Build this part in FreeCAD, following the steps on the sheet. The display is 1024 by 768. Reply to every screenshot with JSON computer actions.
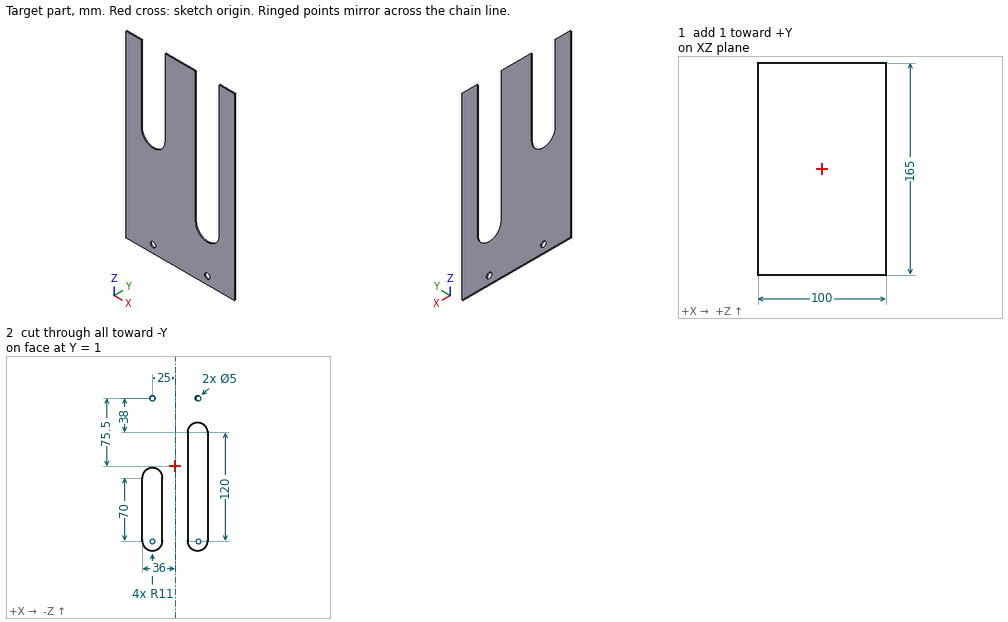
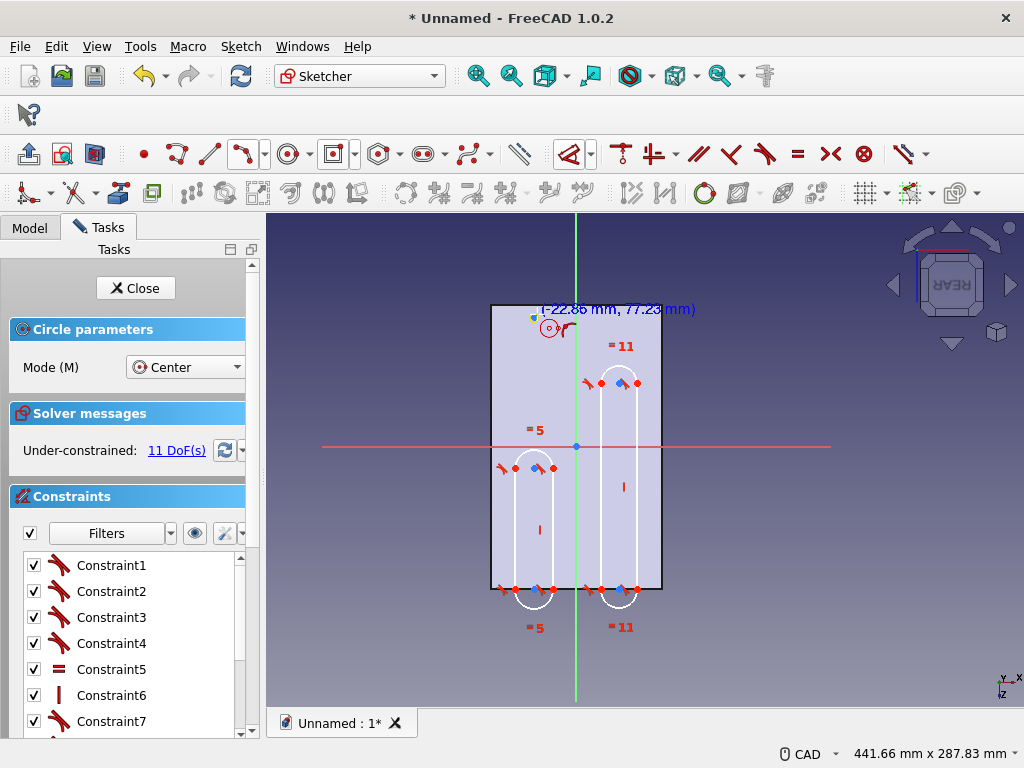
{"action": "scroll", "coordinate": [619, 317], "scroll_direction": "up", "scroll_amount": 9}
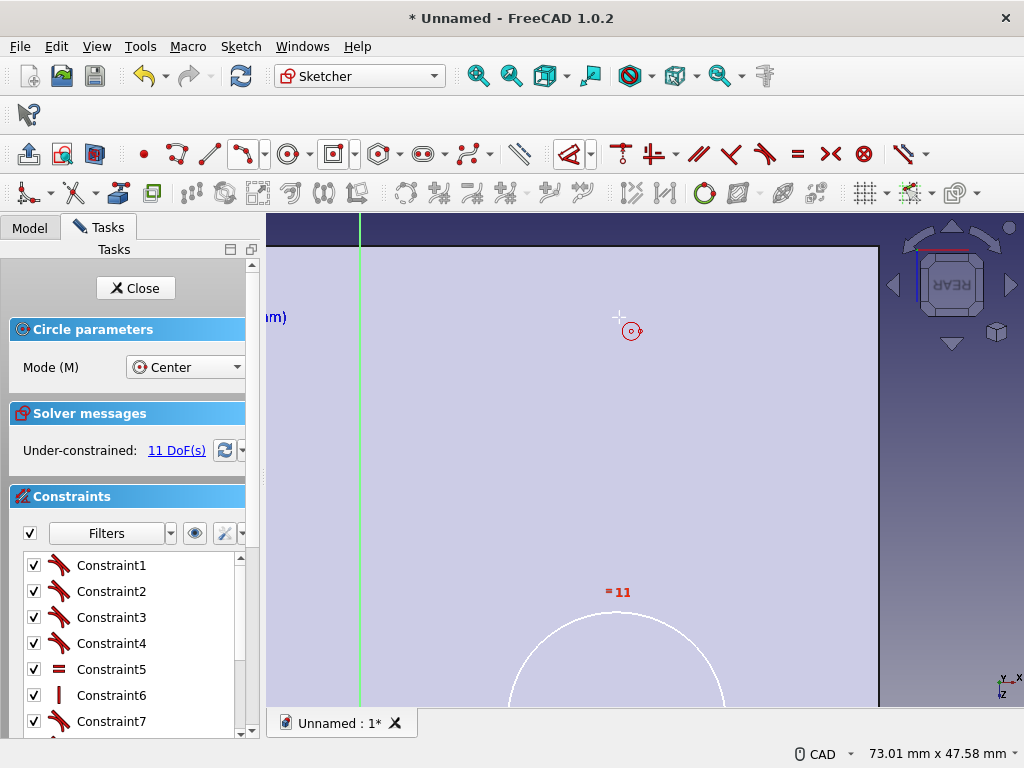
{"action": "scroll", "coordinate": [619, 317], "scroll_direction": "down", "scroll_amount": 9}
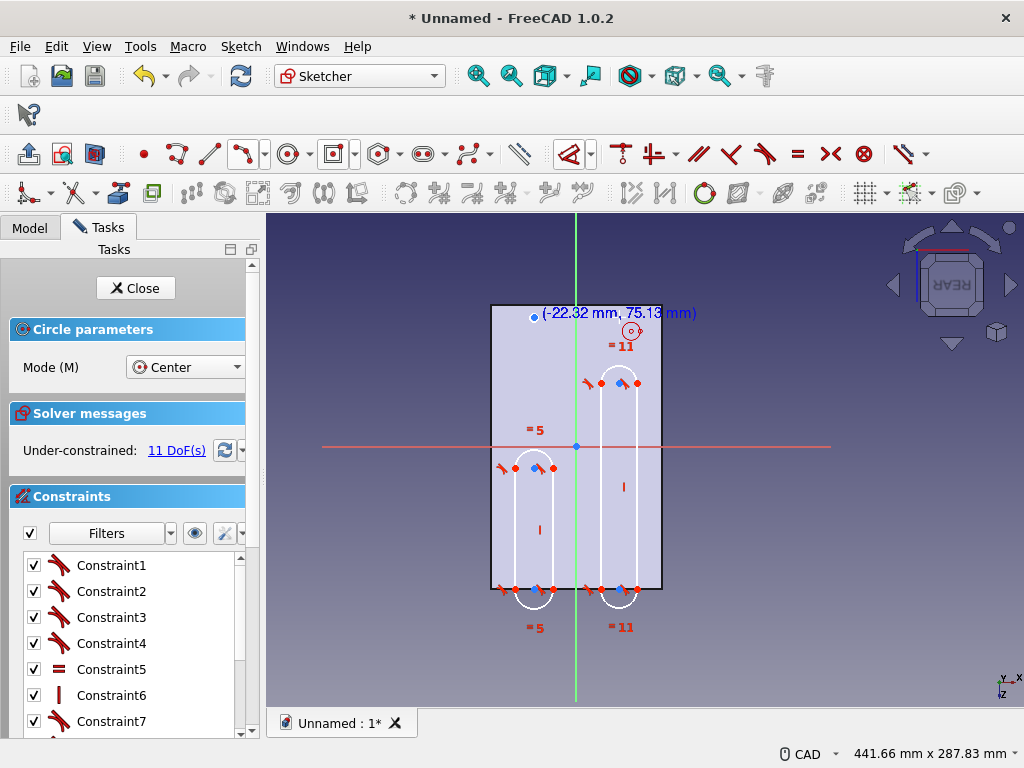
{"action": "left_click", "coordinate": [619, 317]}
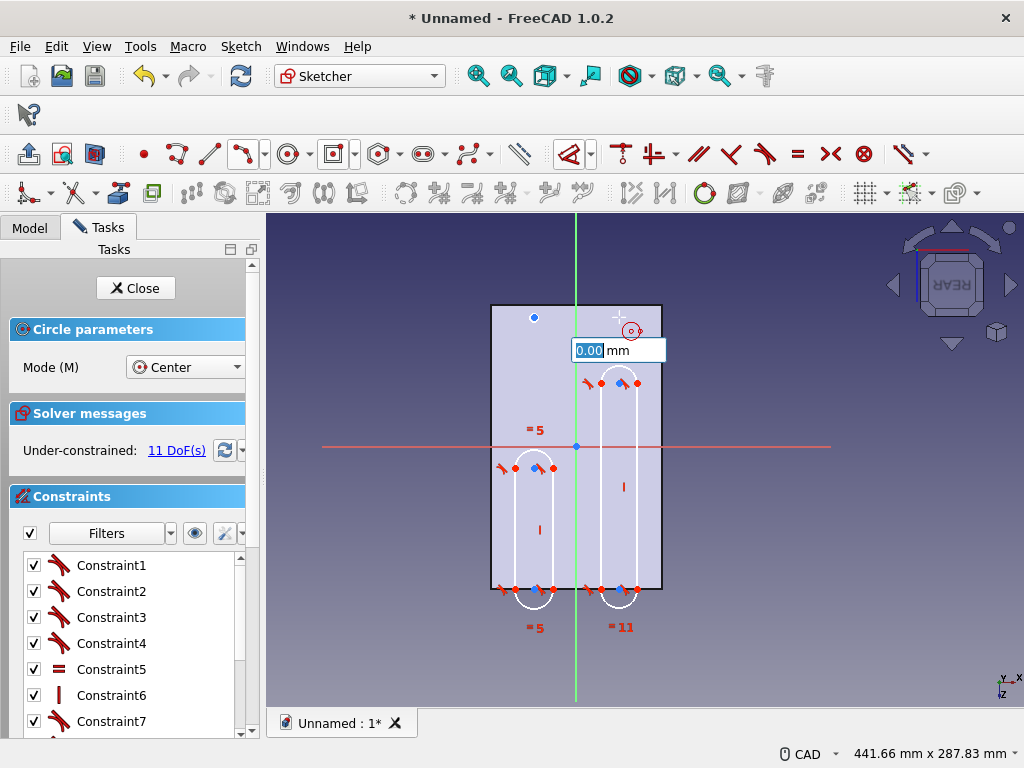
{"action": "scroll", "coordinate": [622, 314], "scroll_direction": "up", "scroll_amount": 7}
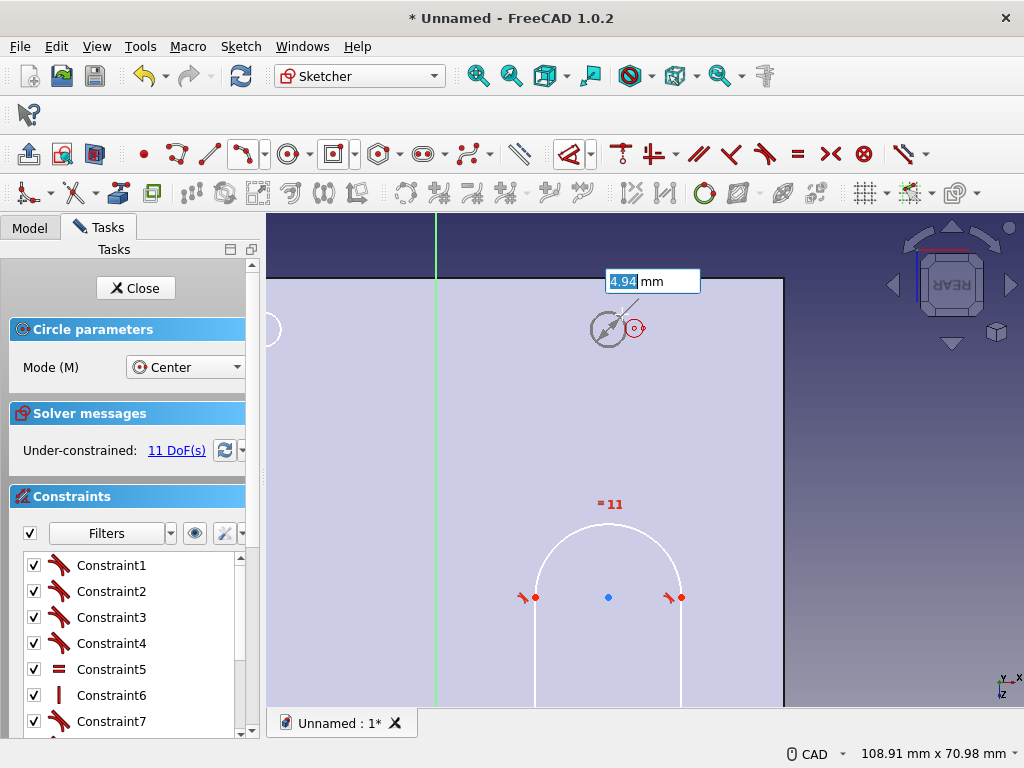
{"action": "left_click", "coordinate": [622, 315]}
{"action": "key", "text": "Escape"}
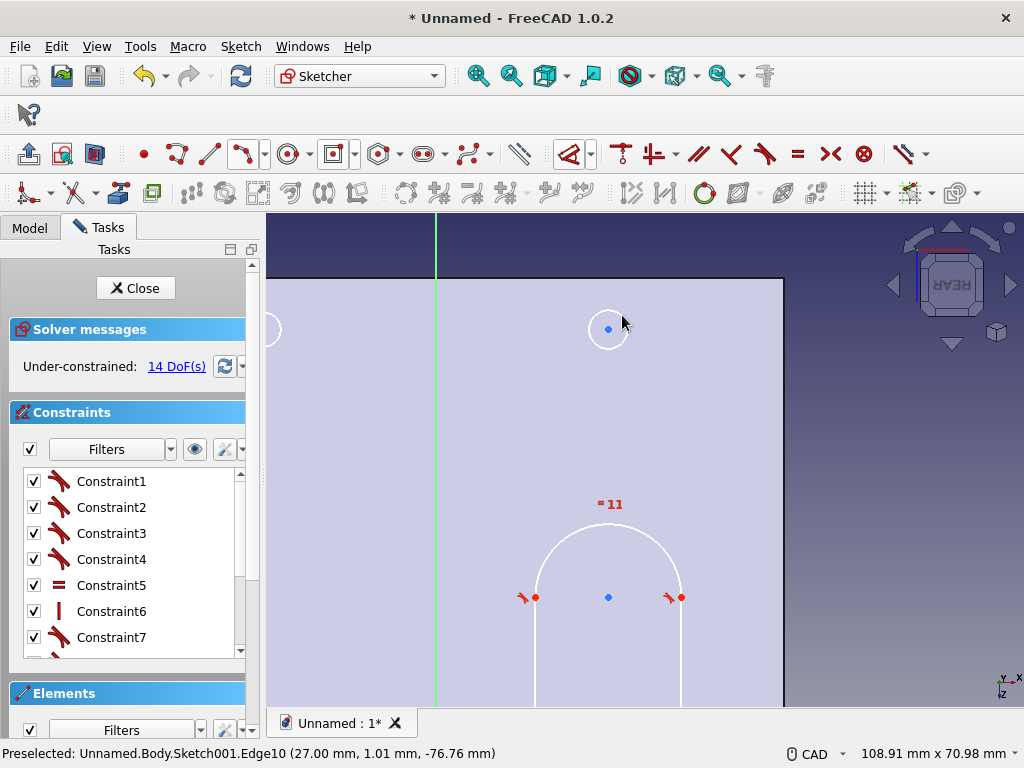
{"action": "scroll", "coordinate": [622, 314], "scroll_direction": "down", "scroll_amount": 7}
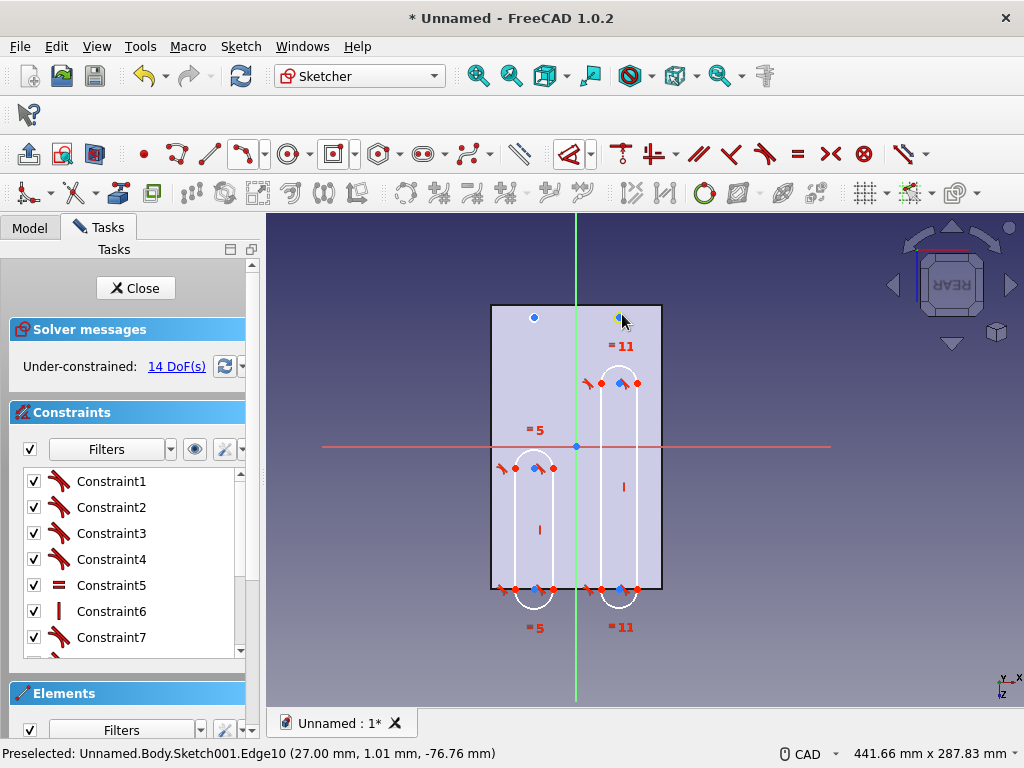
{"action": "left_click", "coordinate": [523, 605]}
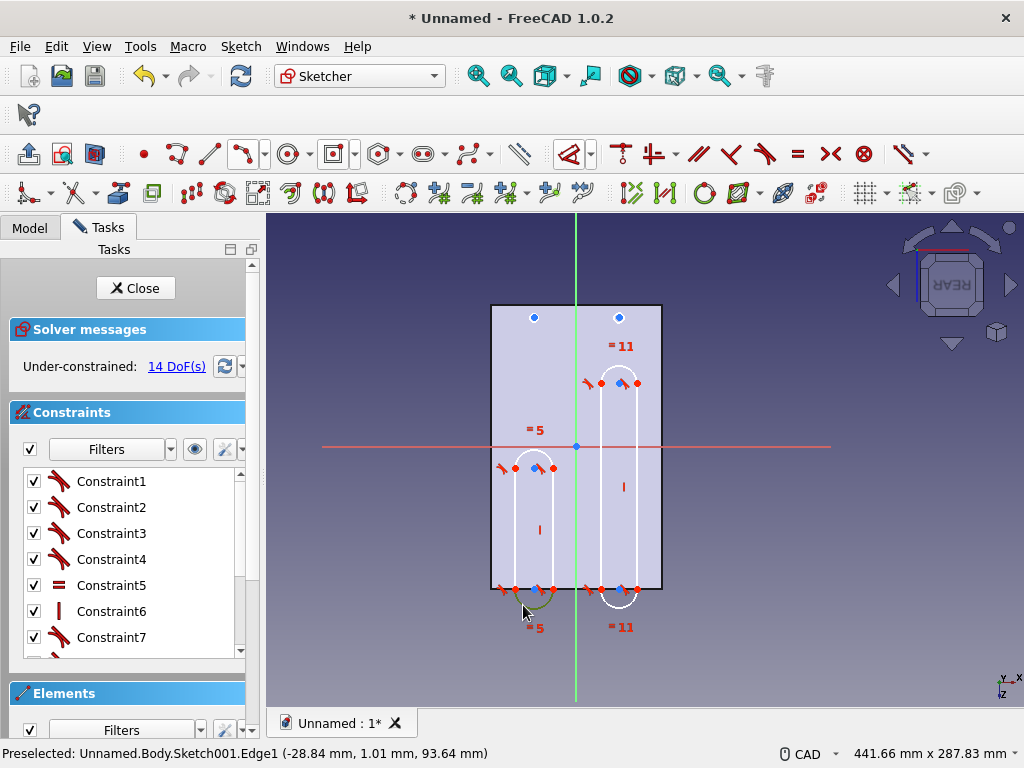
{"action": "left_click", "coordinate": [608, 605]}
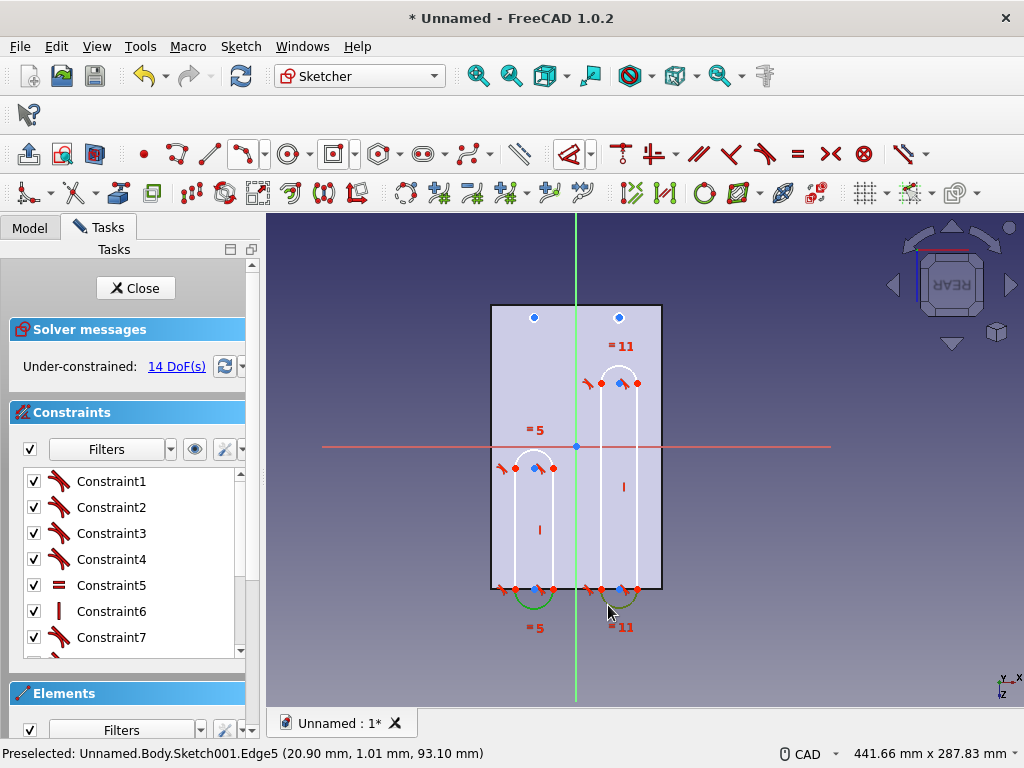
{"action": "left_click", "coordinate": [798, 154]}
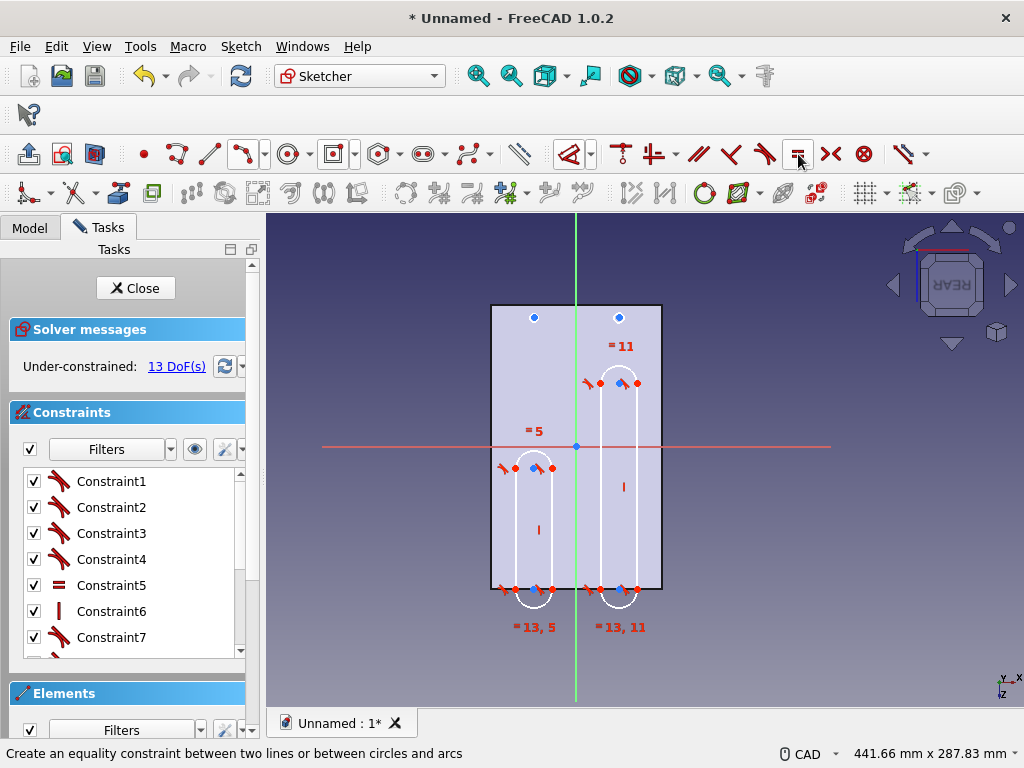
{"action": "scroll", "coordinate": [534, 314], "scroll_direction": "up", "scroll_amount": 6}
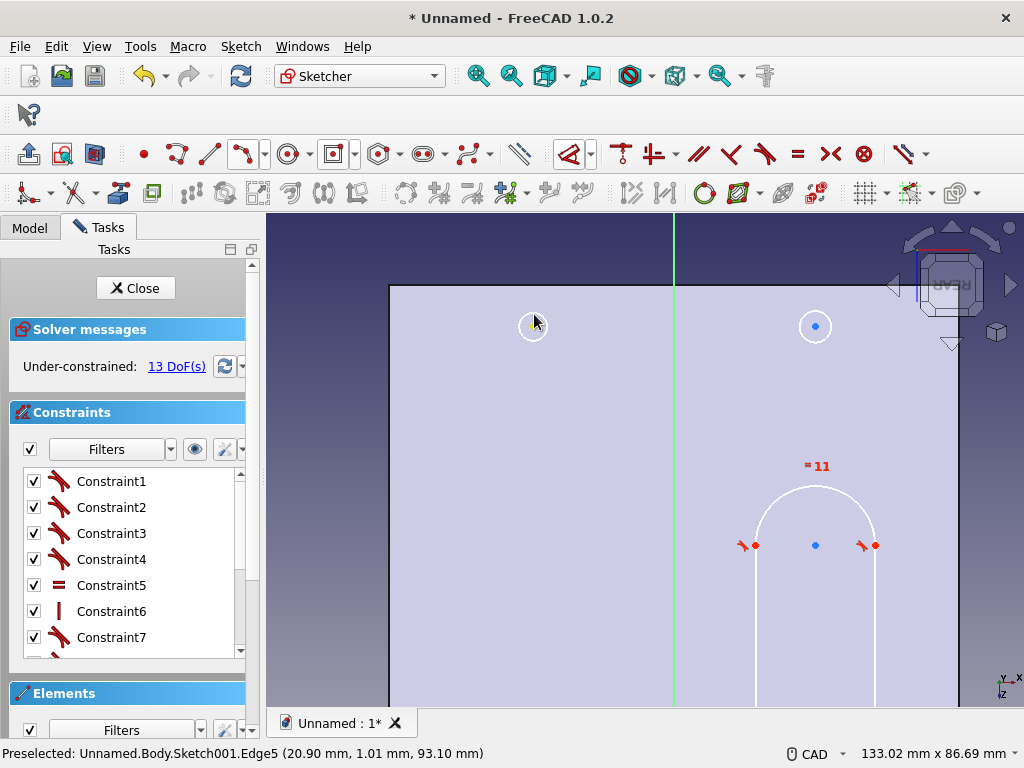
{"action": "left_click", "coordinate": [534, 313]}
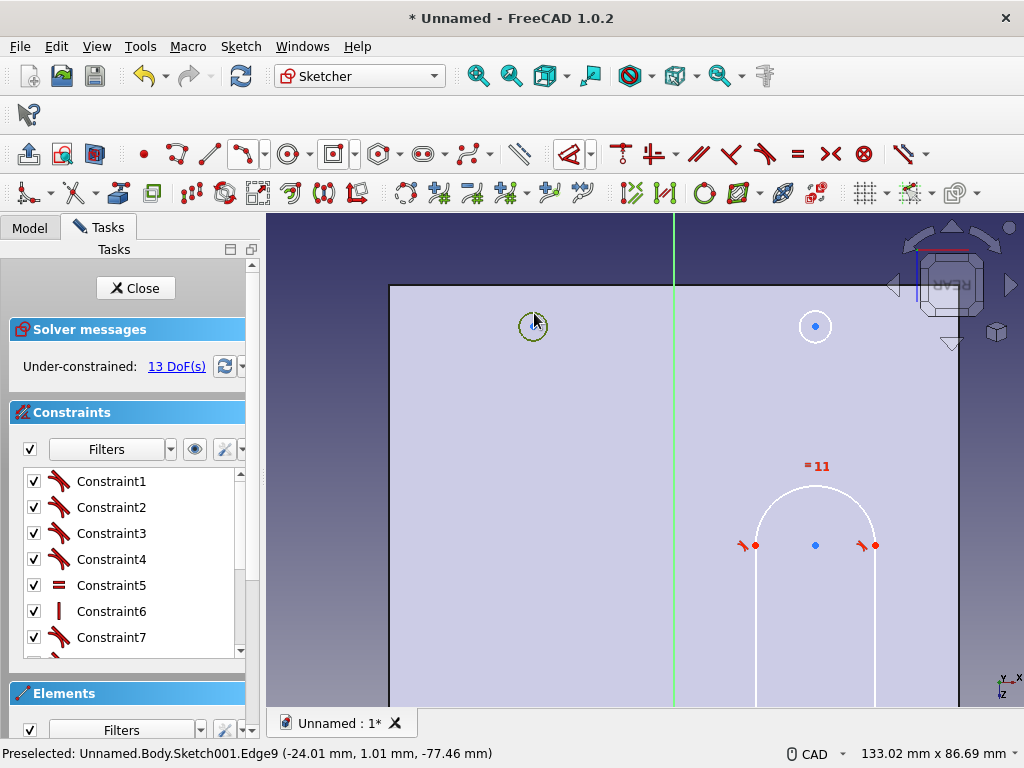
{"action": "left_click", "coordinate": [826, 316]}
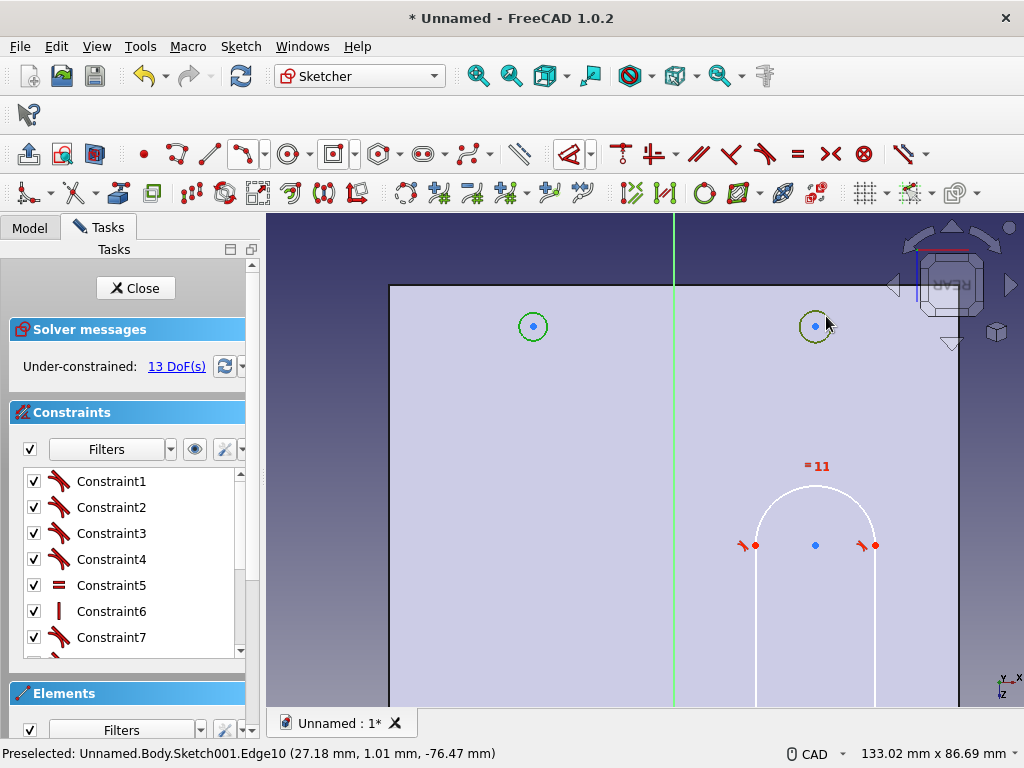
{"action": "left_click", "coordinate": [798, 154]}